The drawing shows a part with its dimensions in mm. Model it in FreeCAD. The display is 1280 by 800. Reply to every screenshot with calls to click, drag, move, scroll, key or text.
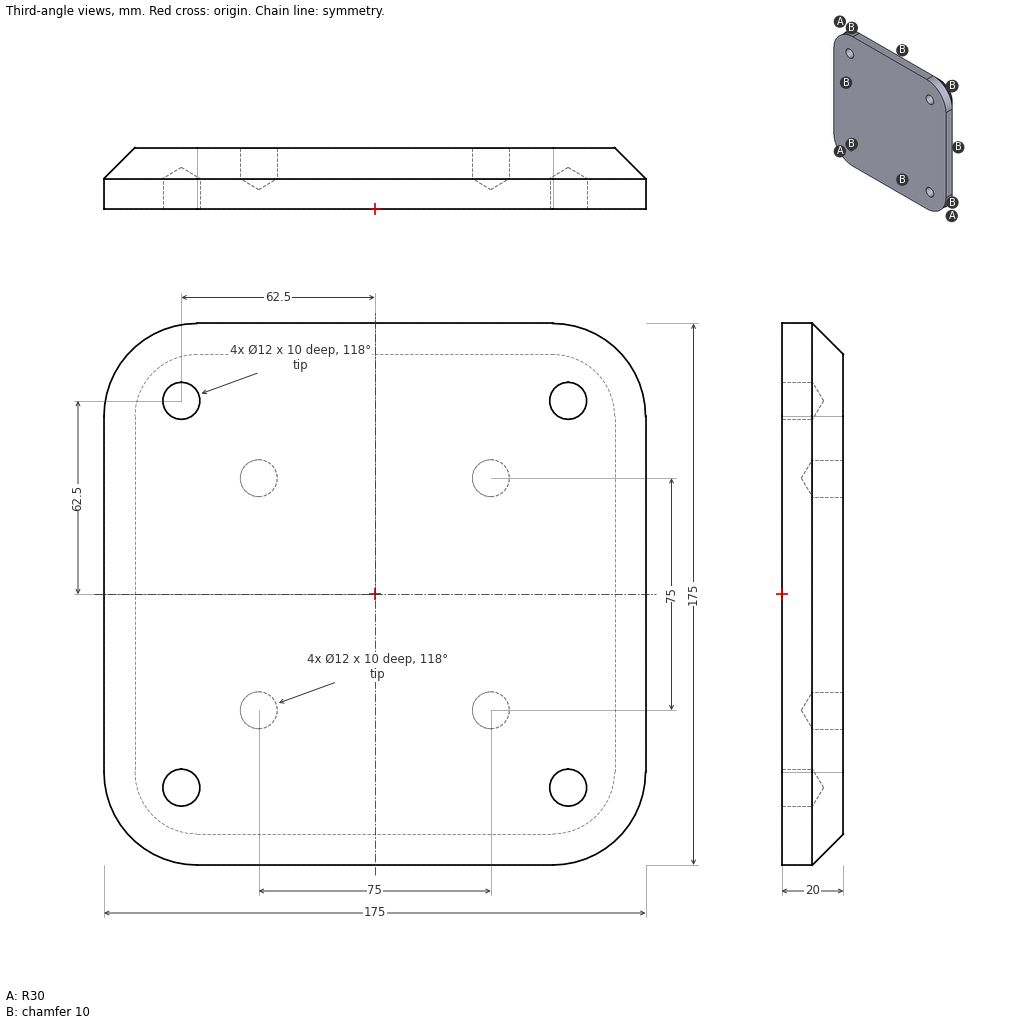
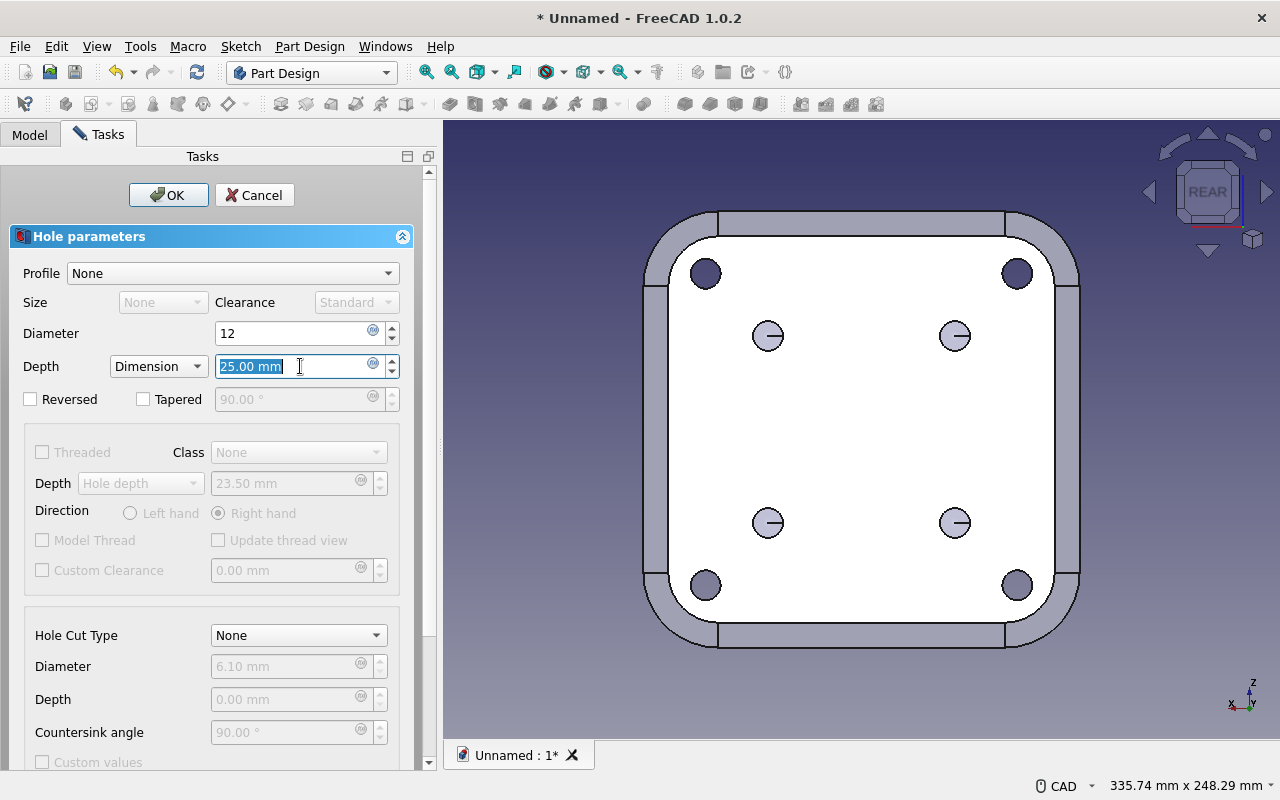
text(10)
key(Tab)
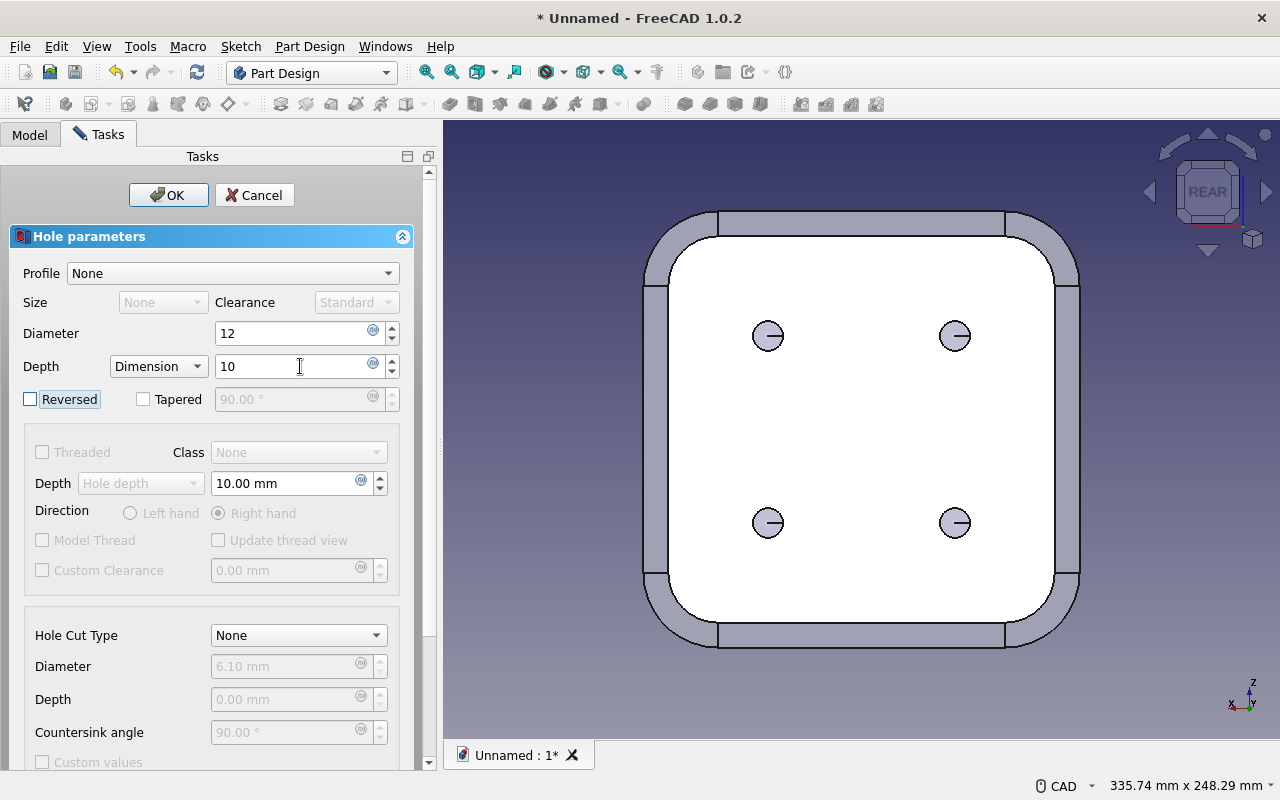
click(169, 195)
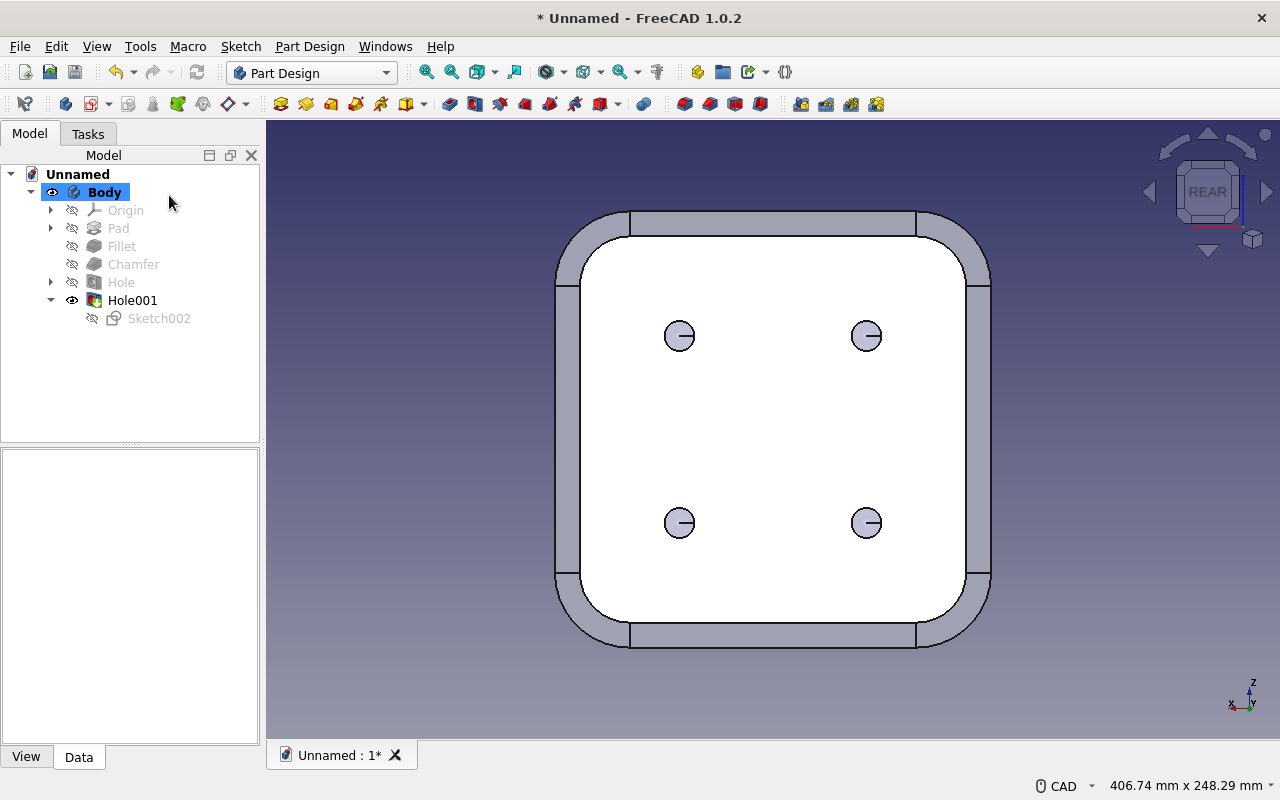
key(0)